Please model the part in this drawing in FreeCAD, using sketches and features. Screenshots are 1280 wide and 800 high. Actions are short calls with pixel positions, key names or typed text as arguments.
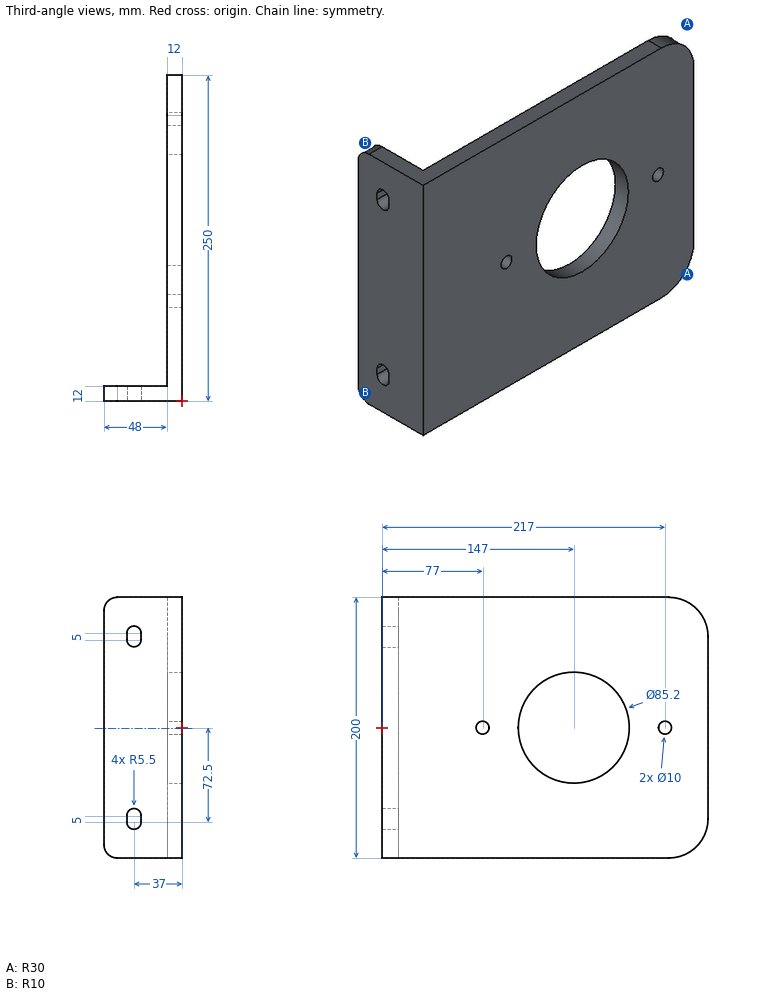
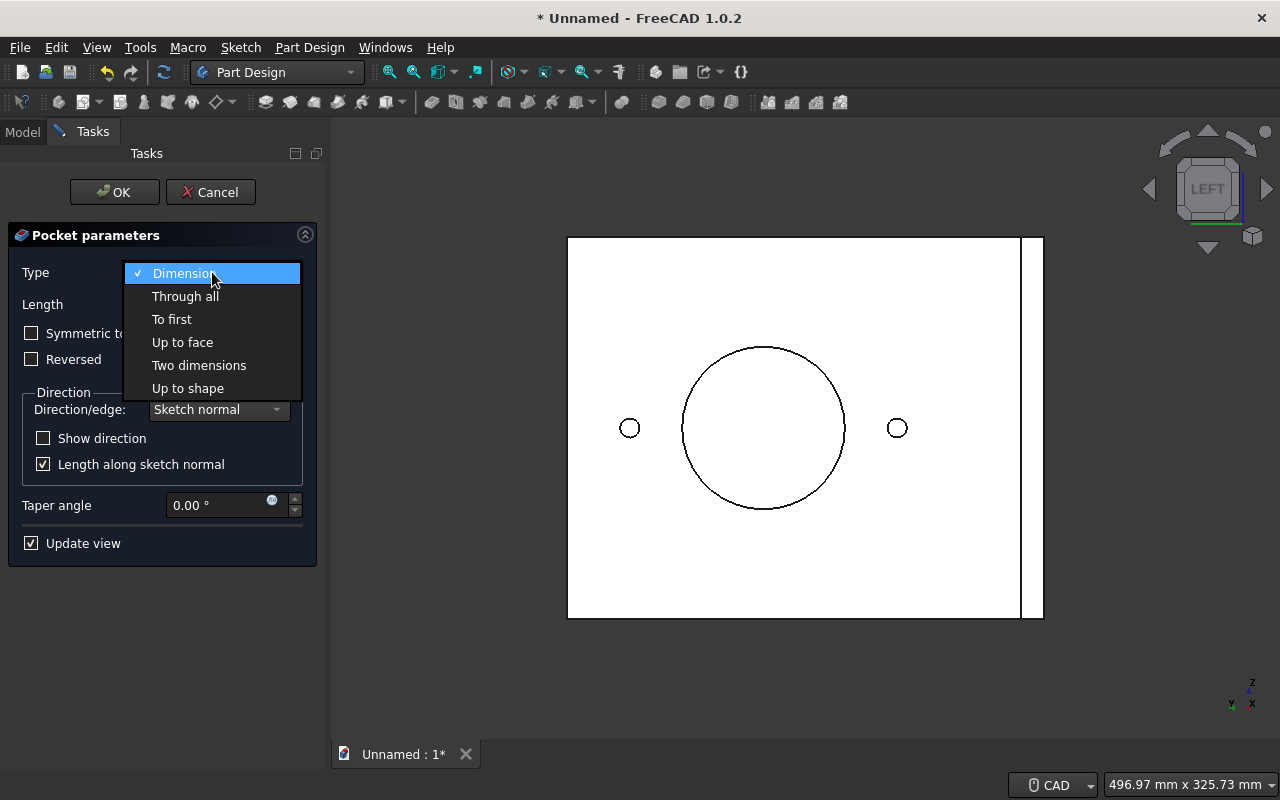
click(212, 296)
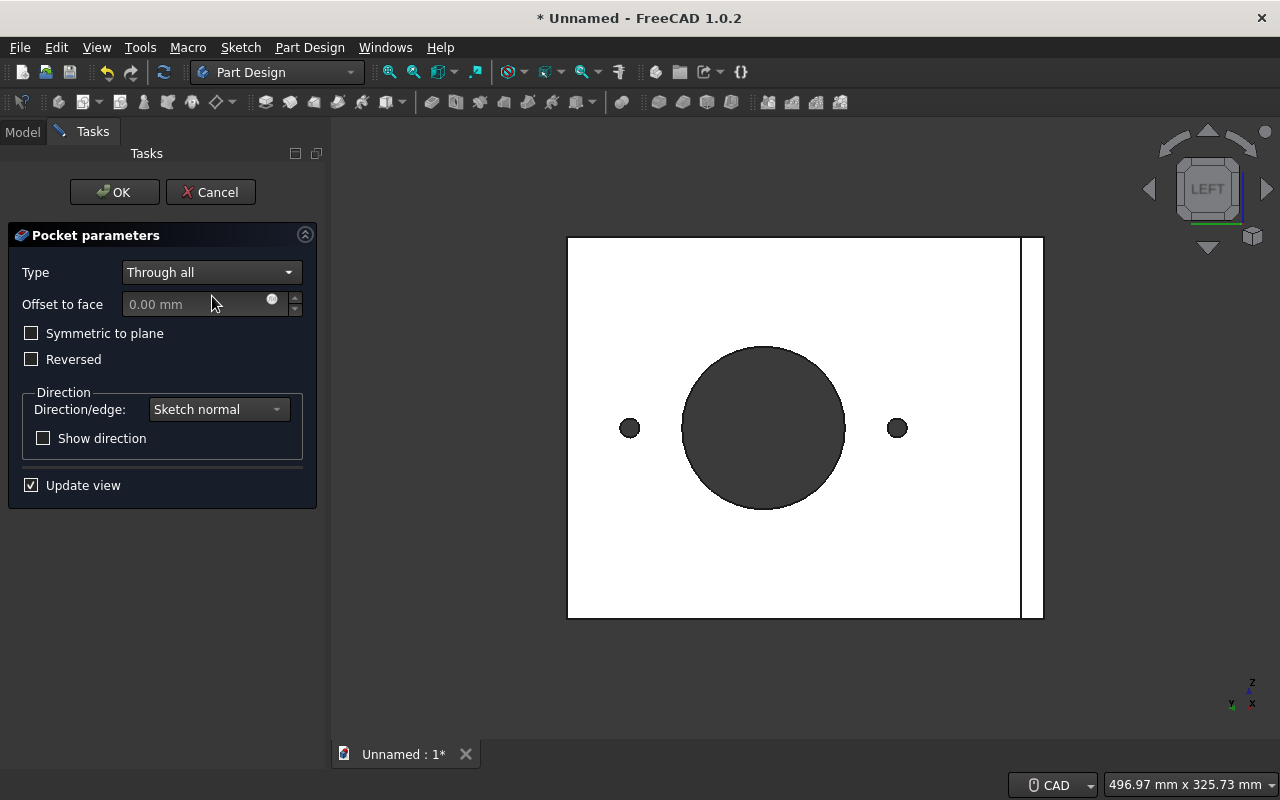
click(115, 192)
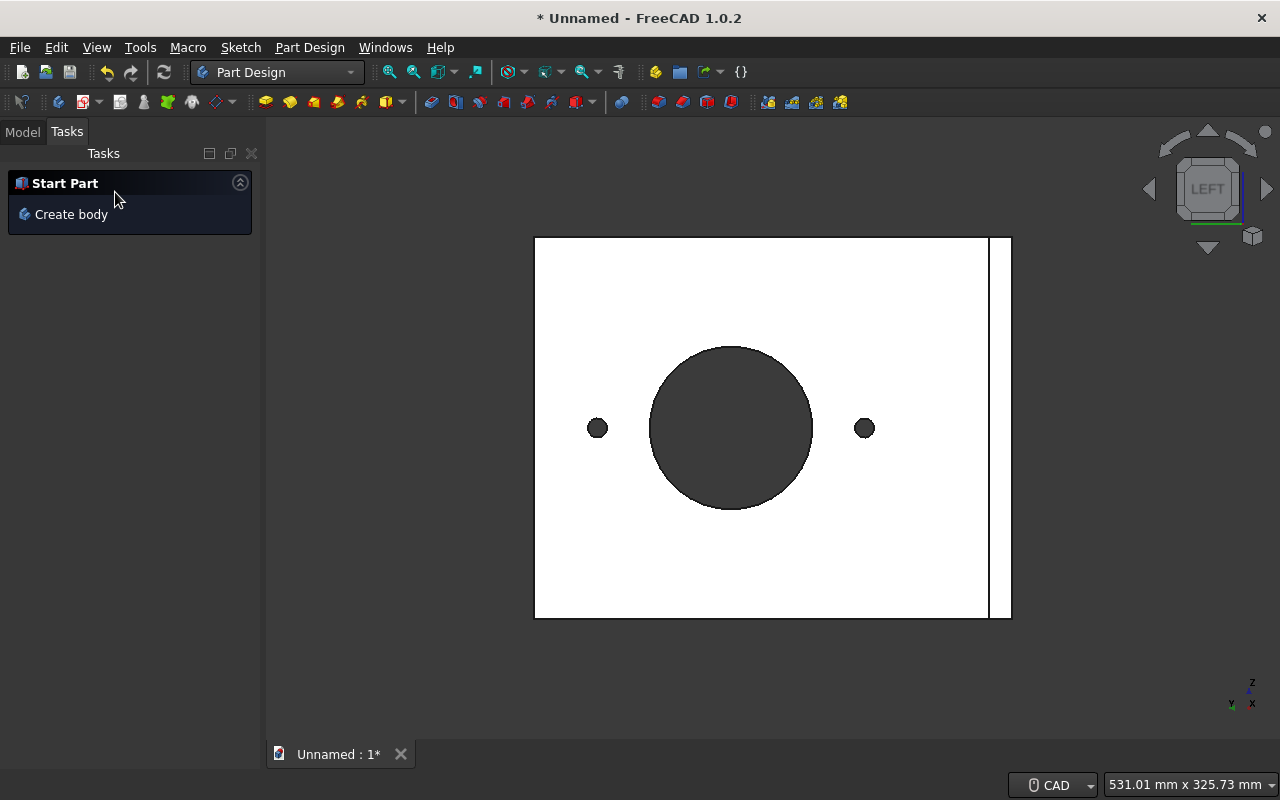
key(0)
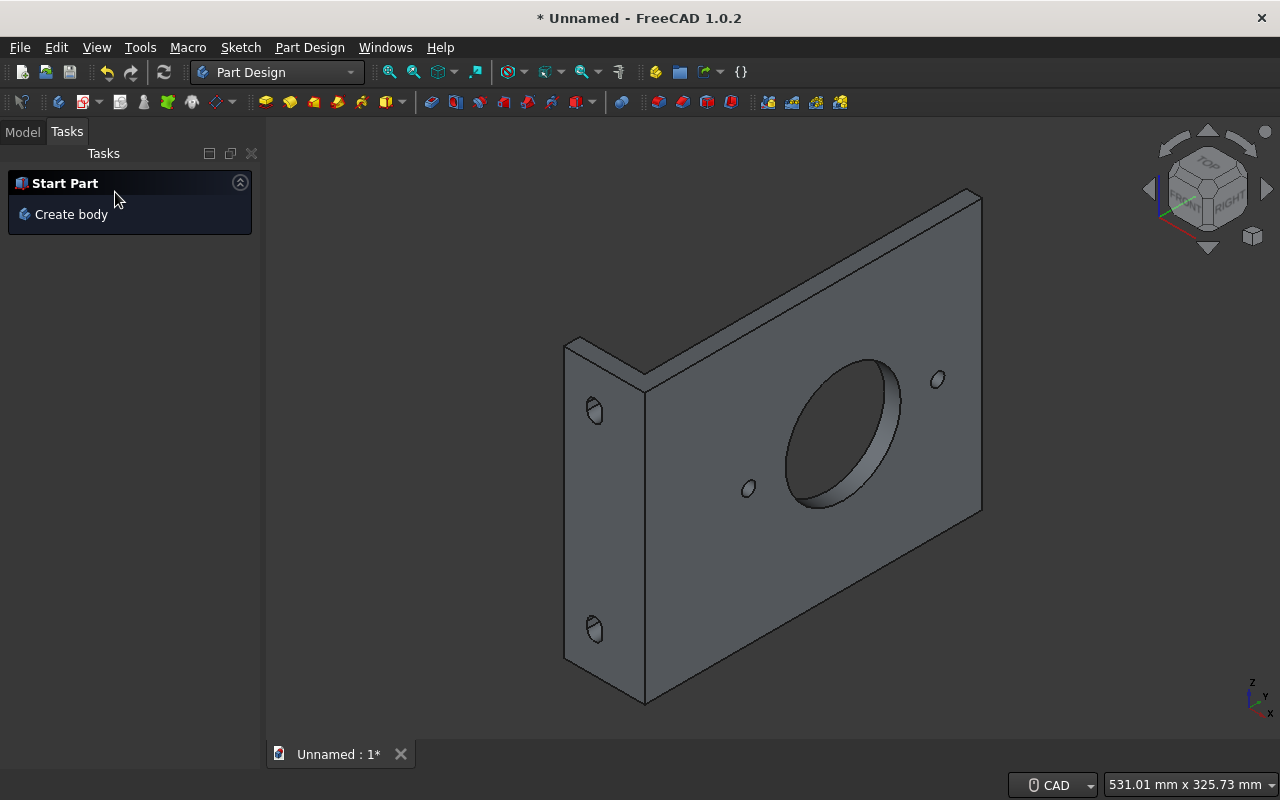
key(2)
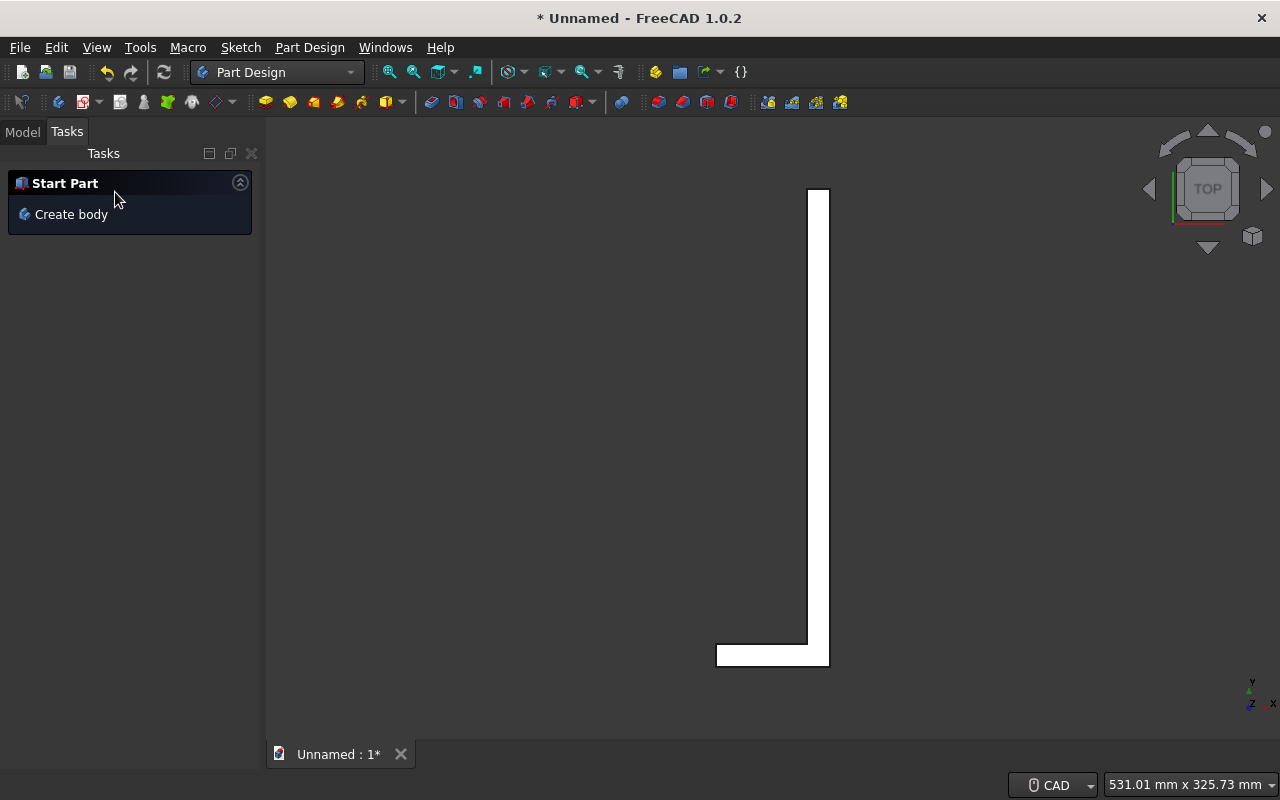
click(819, 188)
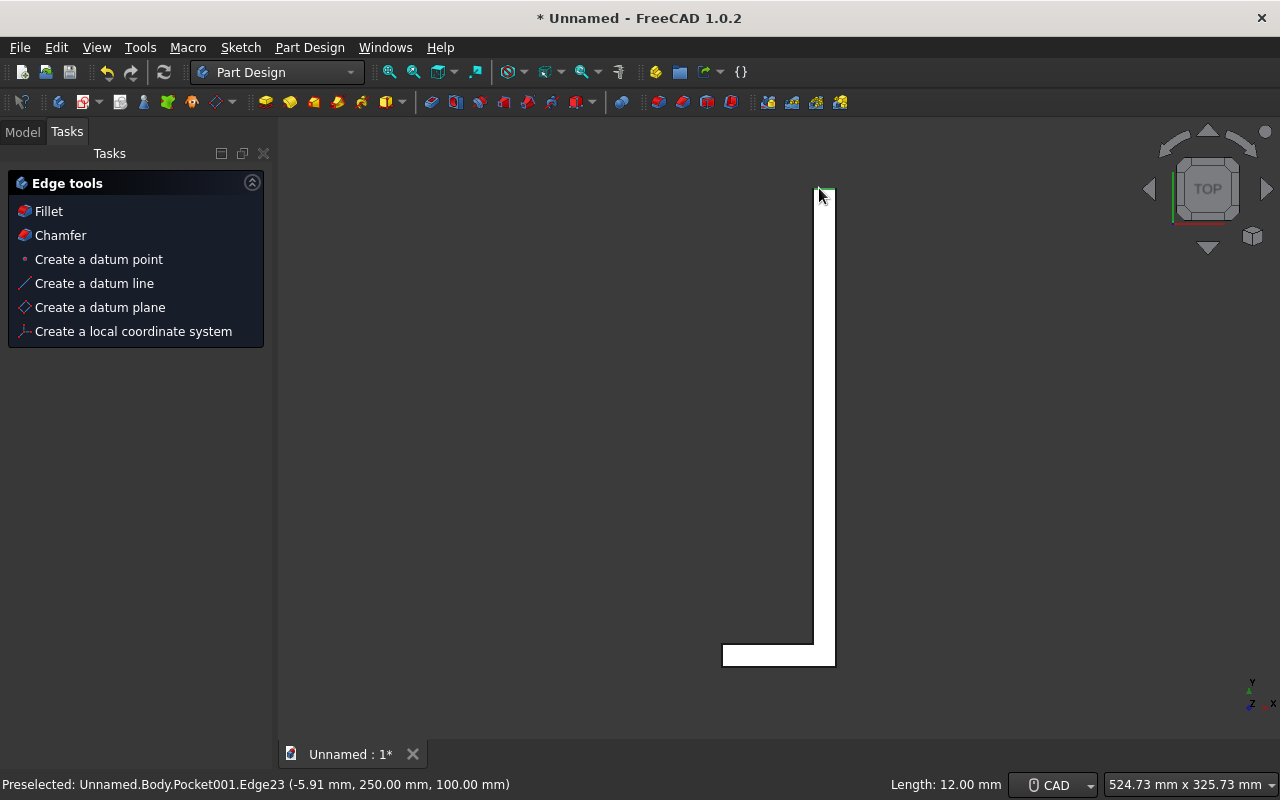
key(1)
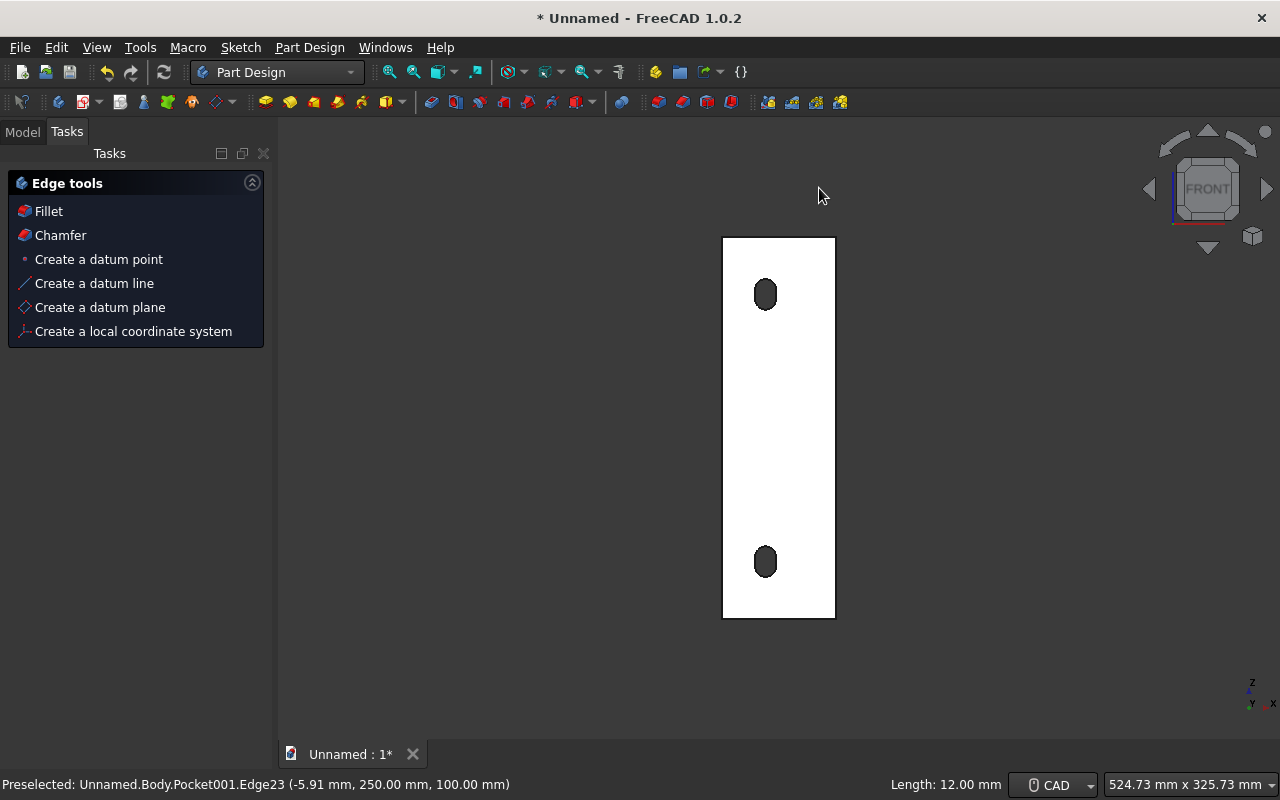
key(3)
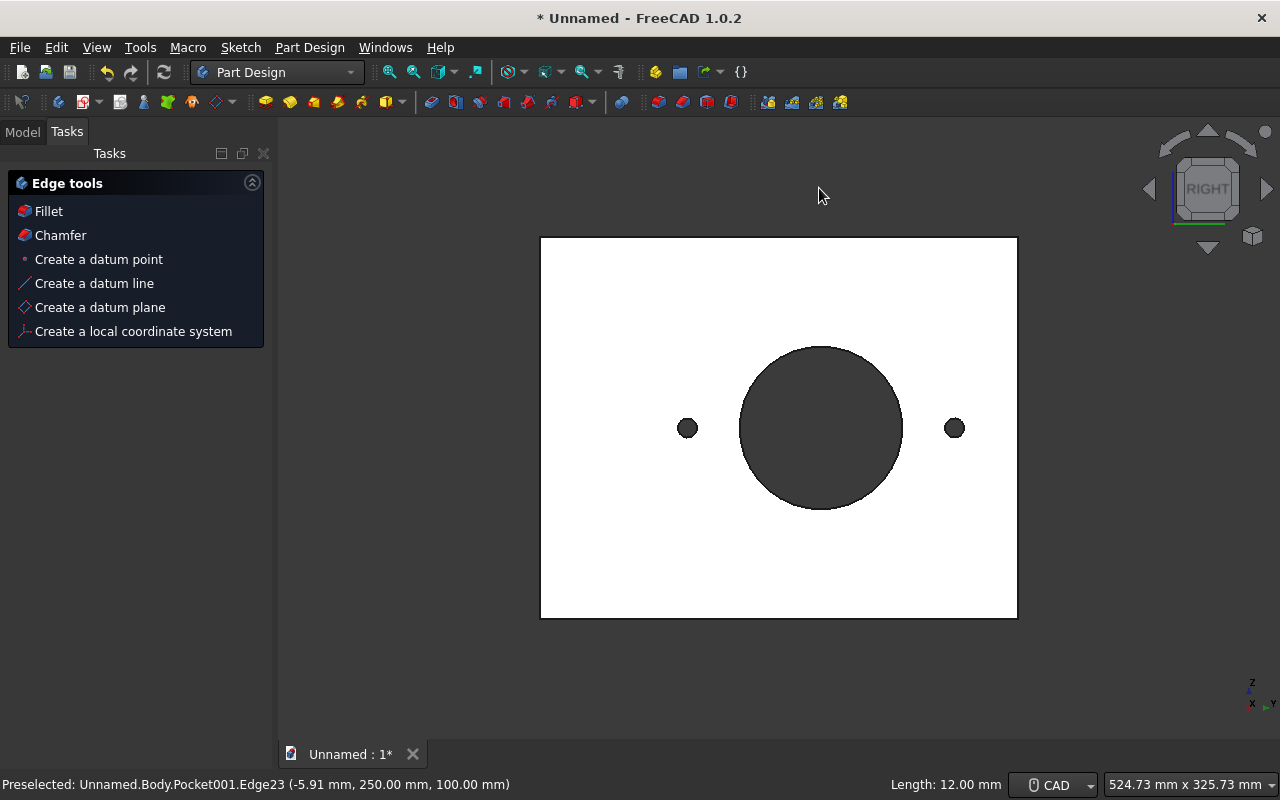
key(5)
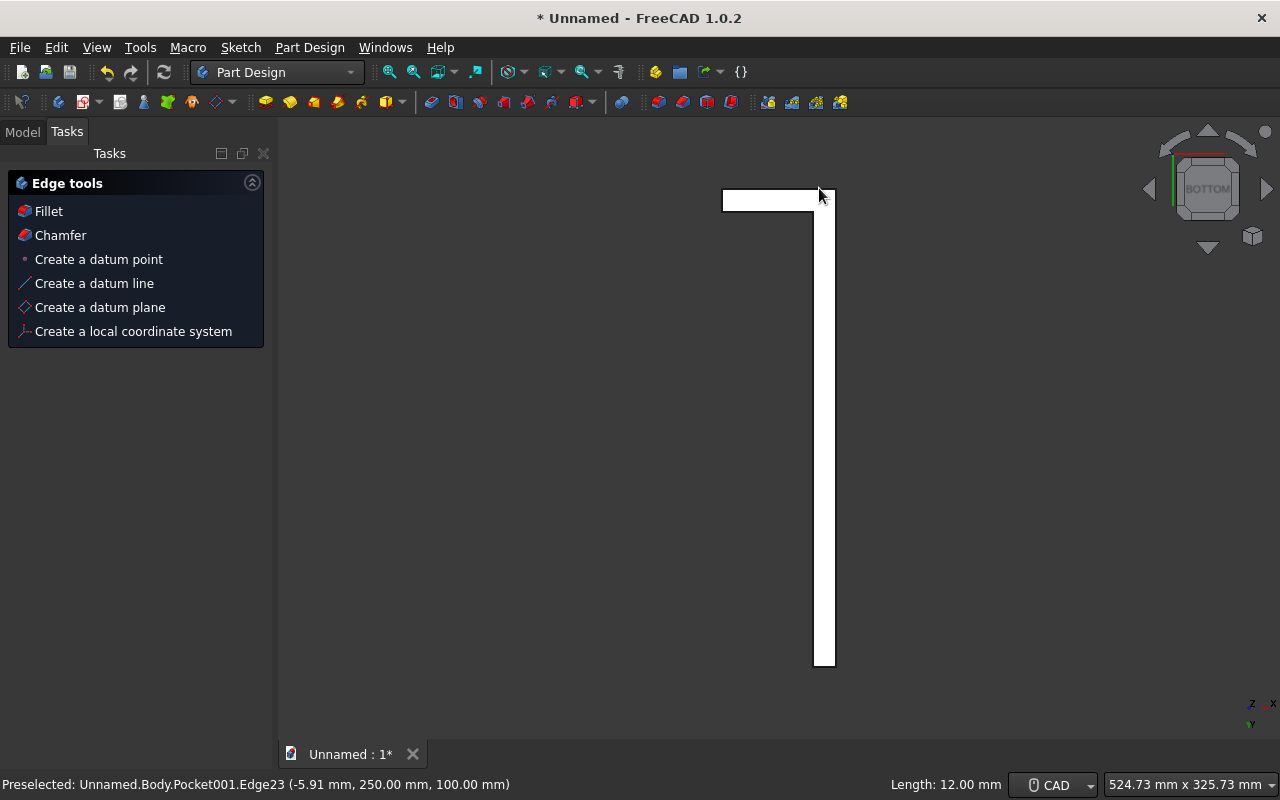
click(825, 666, ctrl)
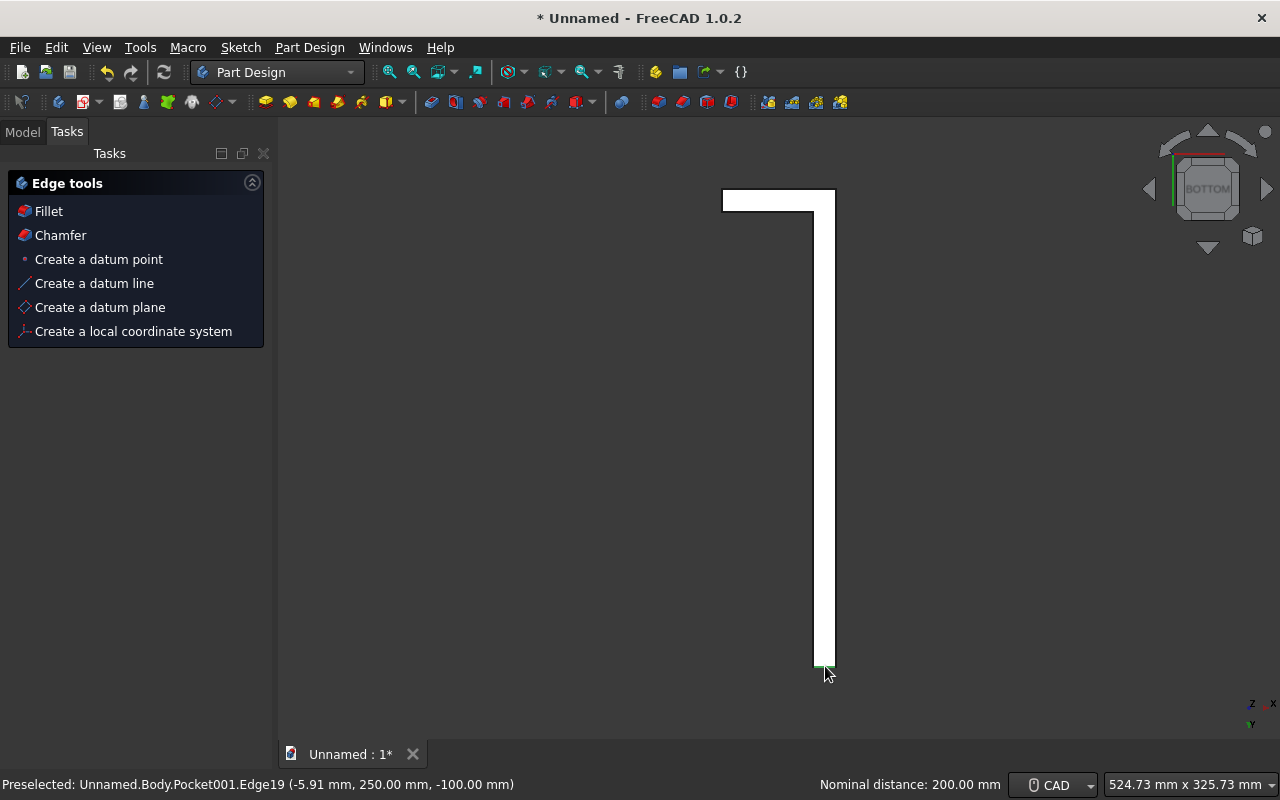
click(660, 102)